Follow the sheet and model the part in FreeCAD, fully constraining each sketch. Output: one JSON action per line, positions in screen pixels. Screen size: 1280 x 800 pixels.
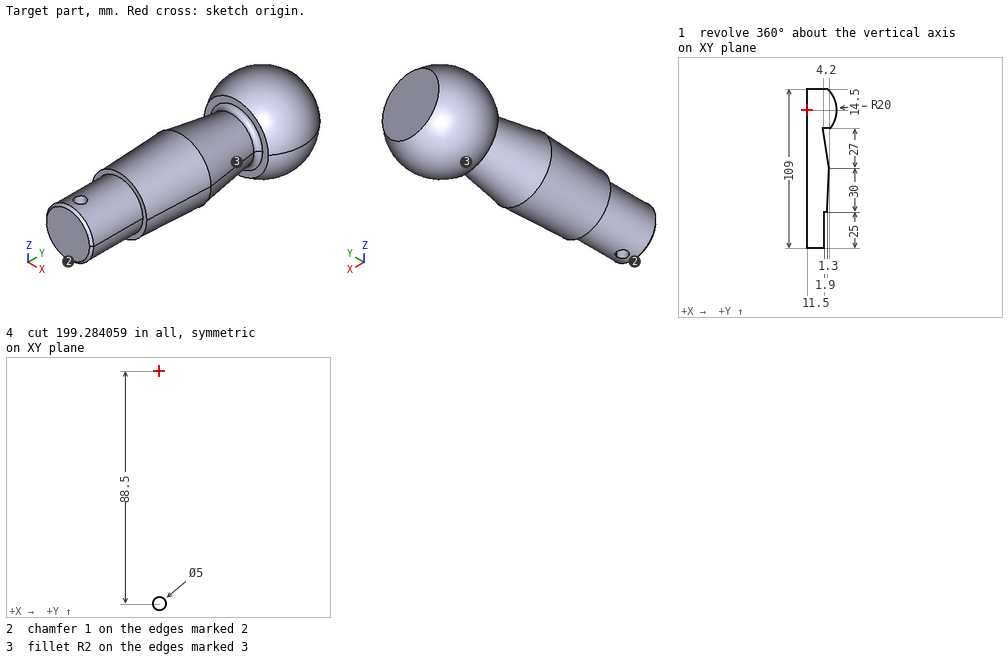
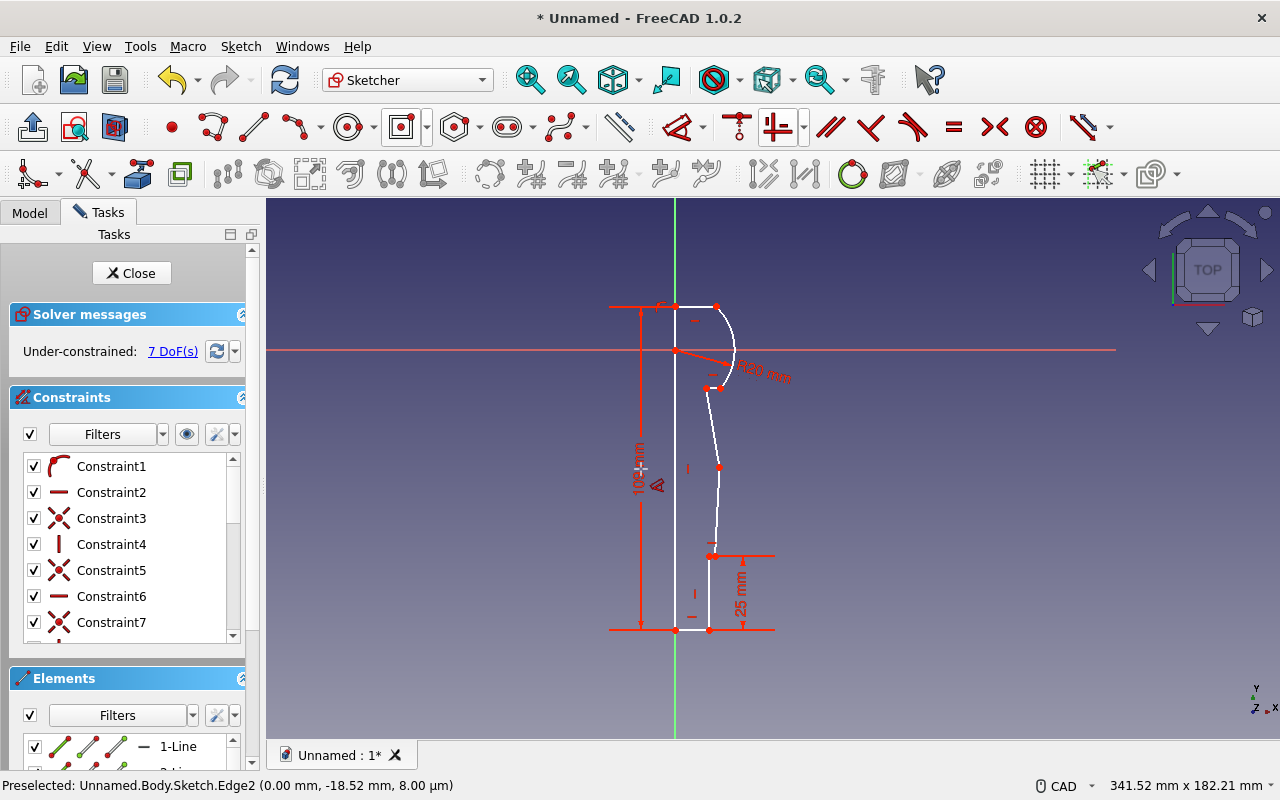
{"action": "scroll", "coordinate": [712, 556], "scroll_direction": "up", "scroll_amount": 10}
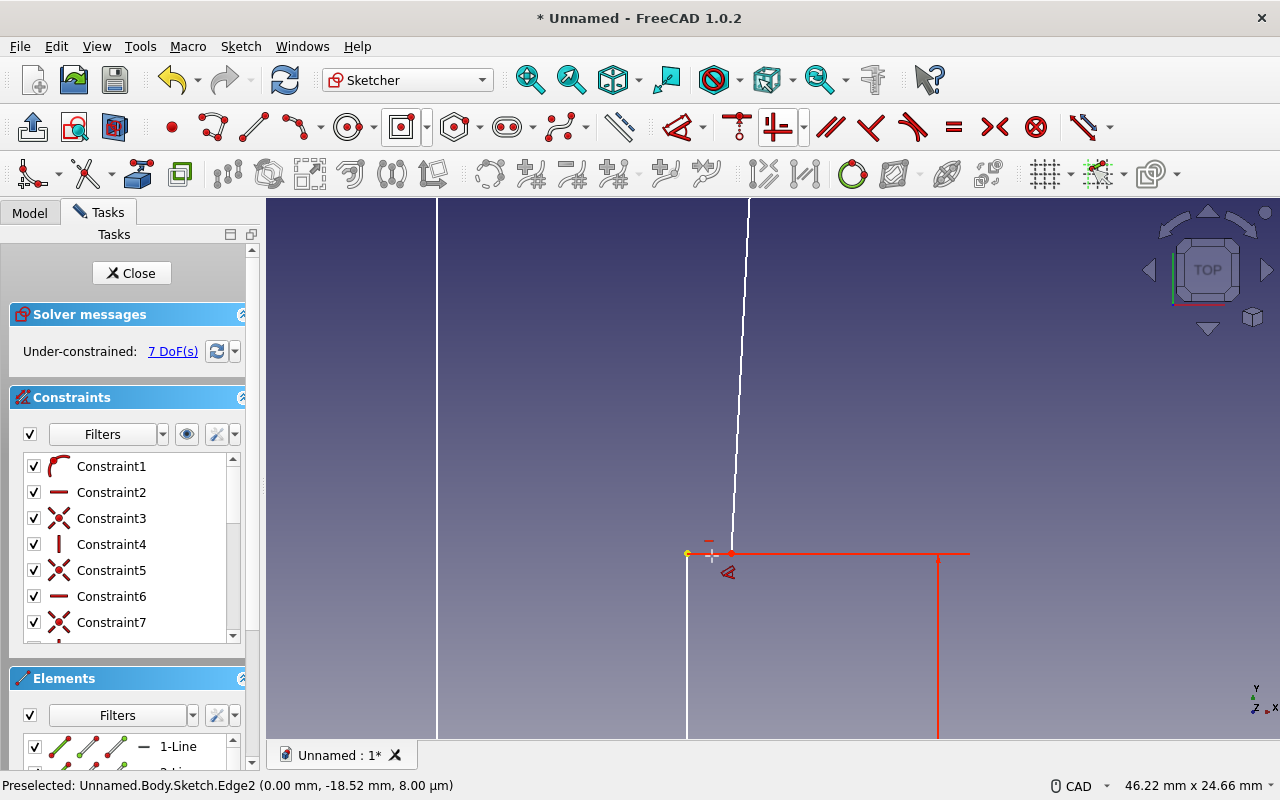
{"action": "left_click", "coordinate": [709, 554]}
{"action": "left_click", "coordinate": [709, 588]}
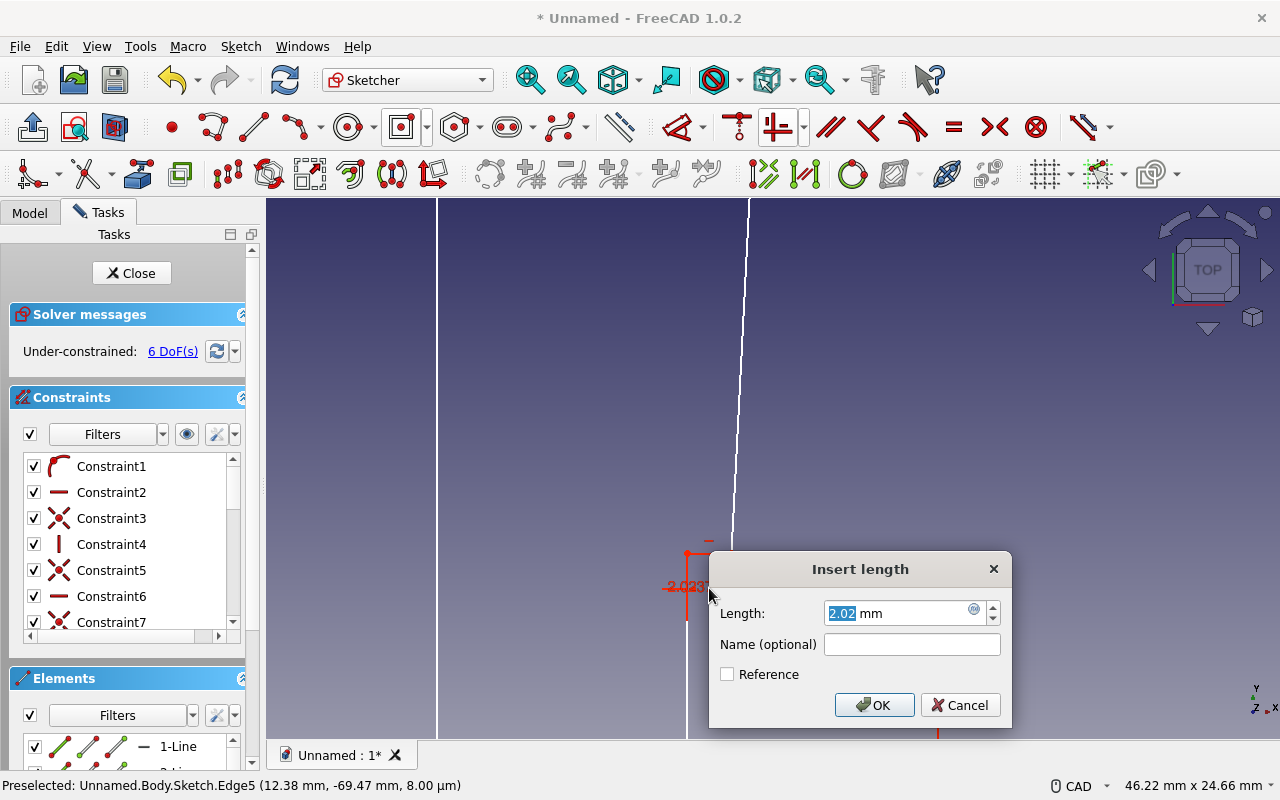
{"action": "type", "text": "1.9"}
{"action": "key", "text": "Return"}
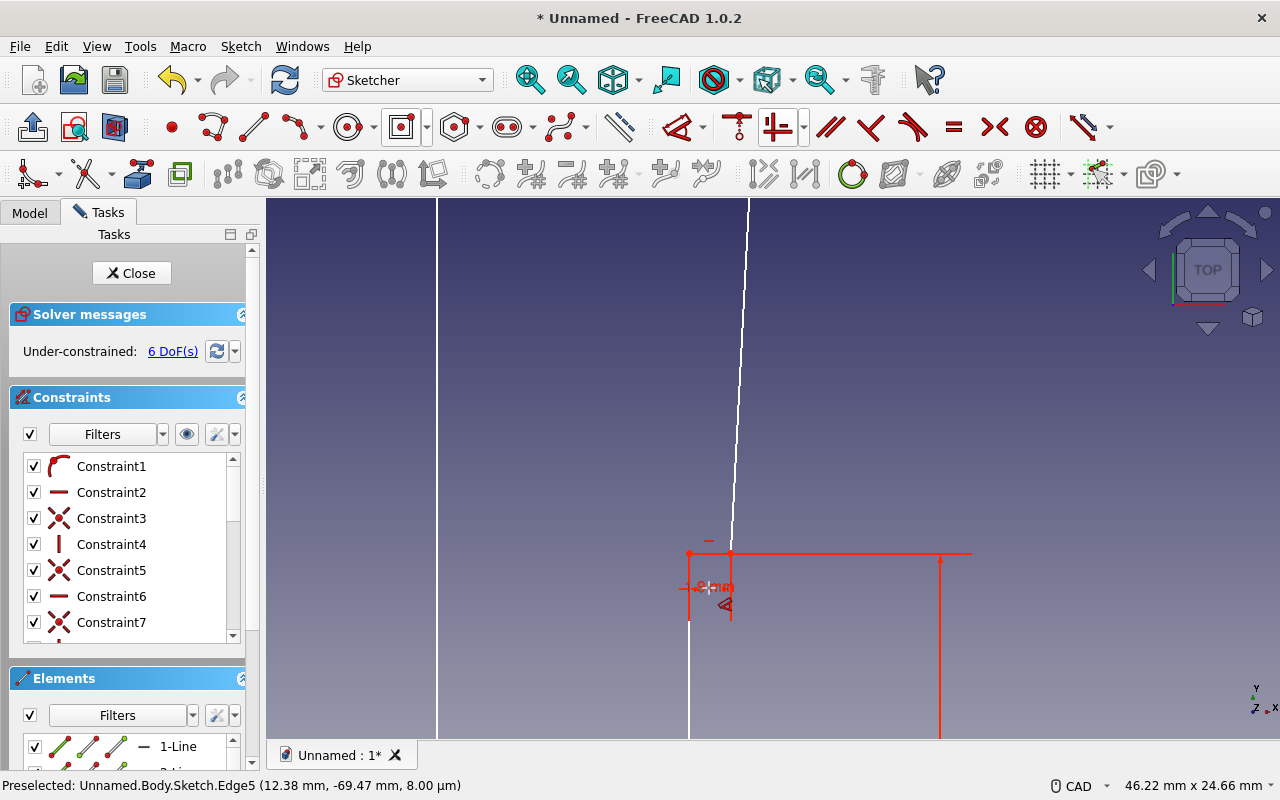
{"action": "scroll", "coordinate": [712, 556], "scroll_direction": "down", "scroll_amount": 10}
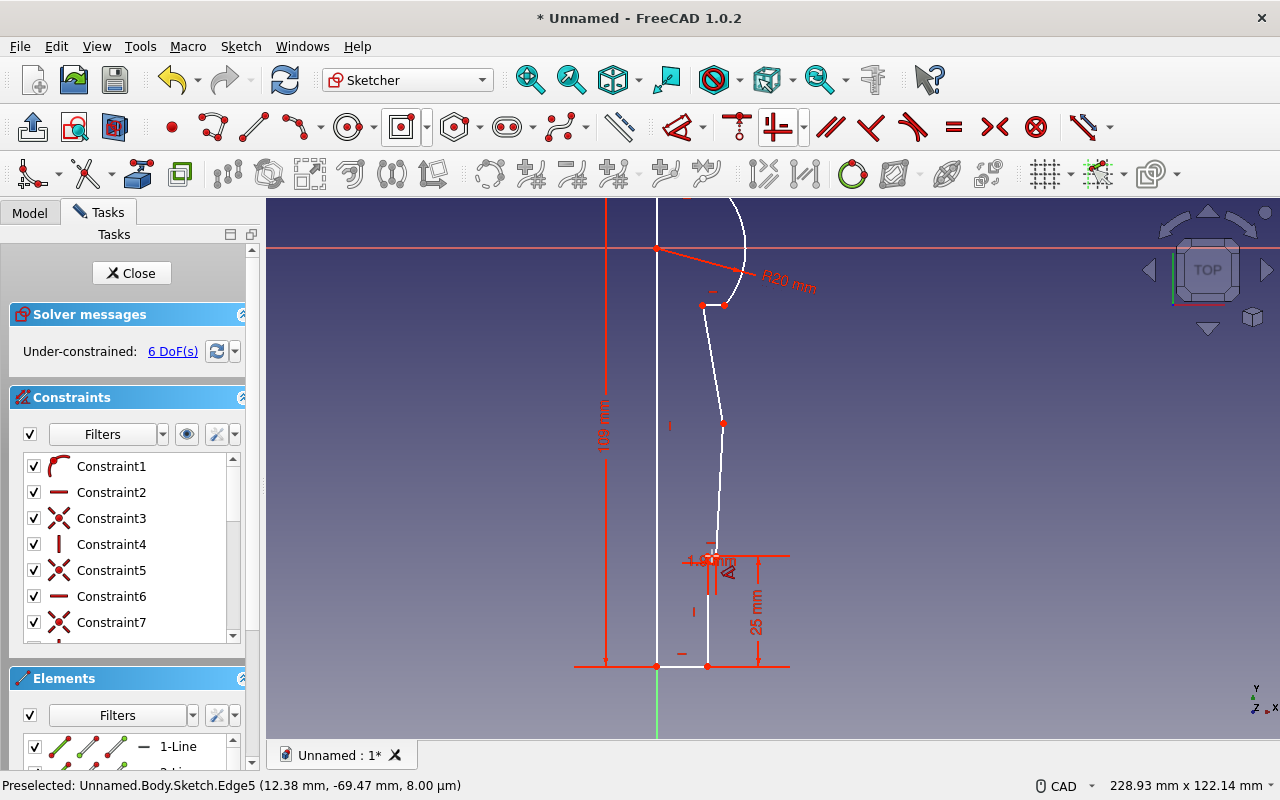
{"action": "left_click", "coordinate": [716, 530]}
{"action": "left_click", "coordinate": [754, 512]}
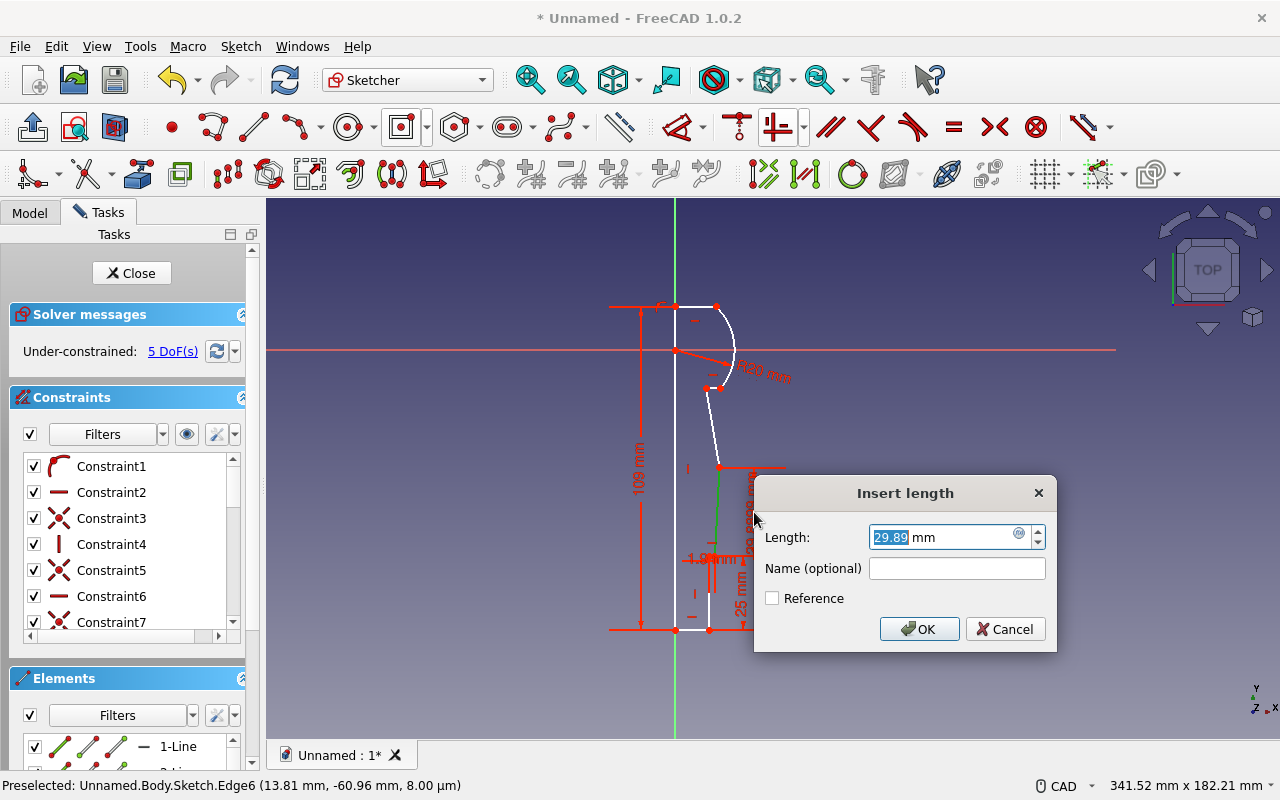
{"action": "type", "text": "30"}
{"action": "key", "text": "Return"}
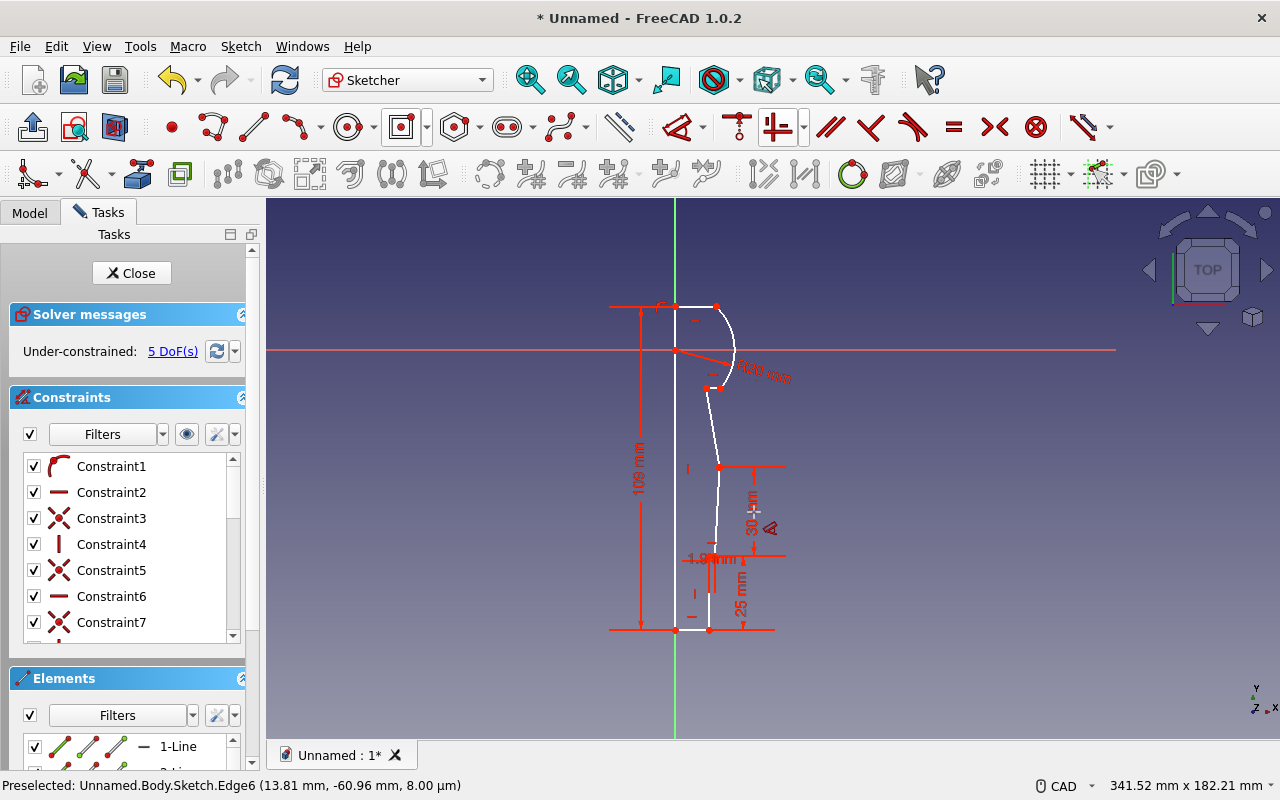
{"action": "left_click", "coordinate": [715, 443]}
{"action": "left_click", "coordinate": [754, 428]}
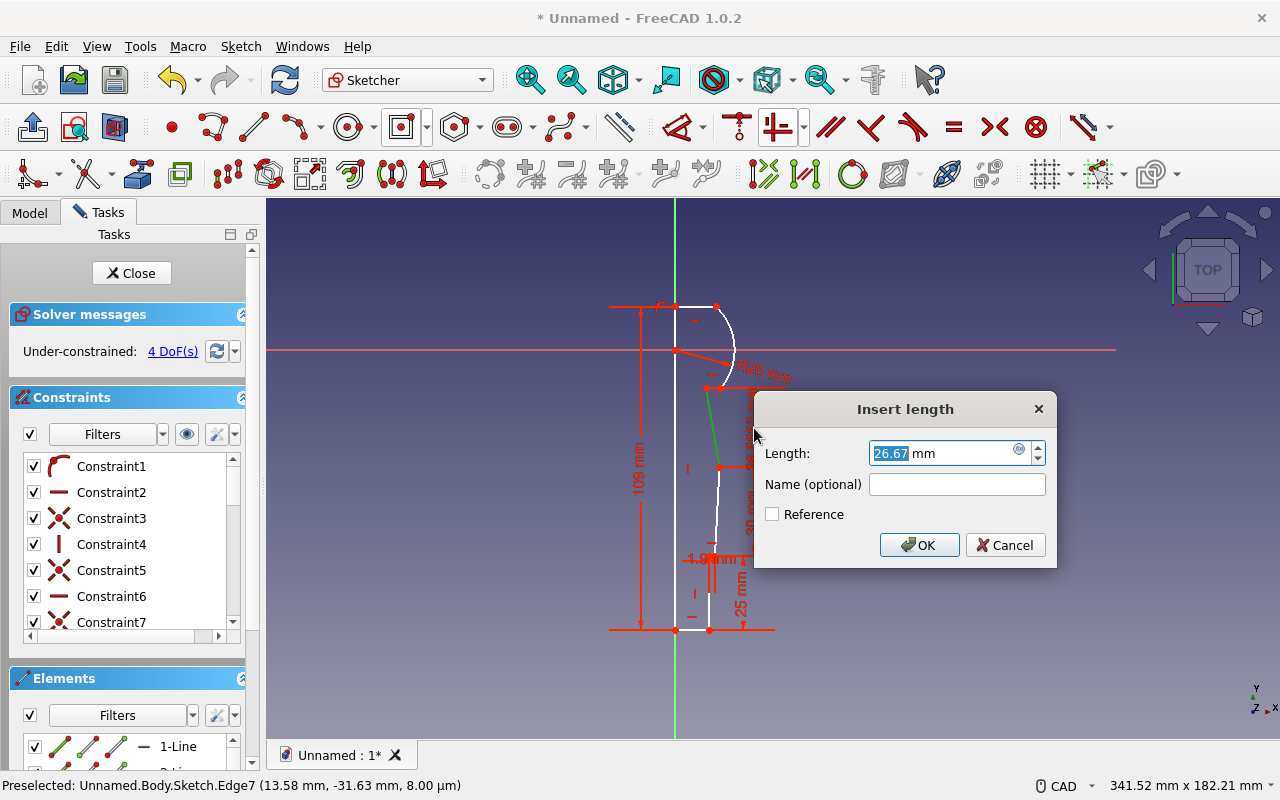
{"action": "type", "text": "27"}
{"action": "key", "text": "Return"}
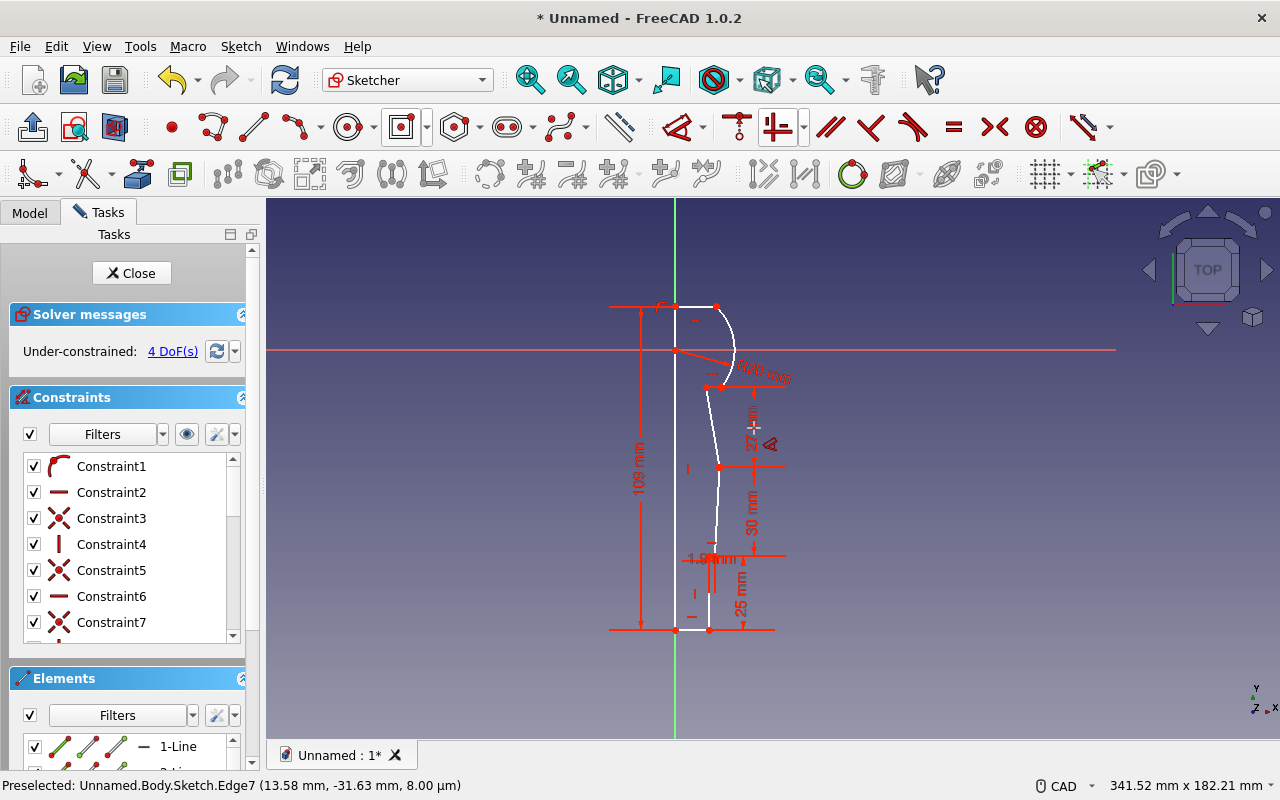
{"action": "scroll", "coordinate": [685, 630], "scroll_direction": "up", "scroll_amount": 2}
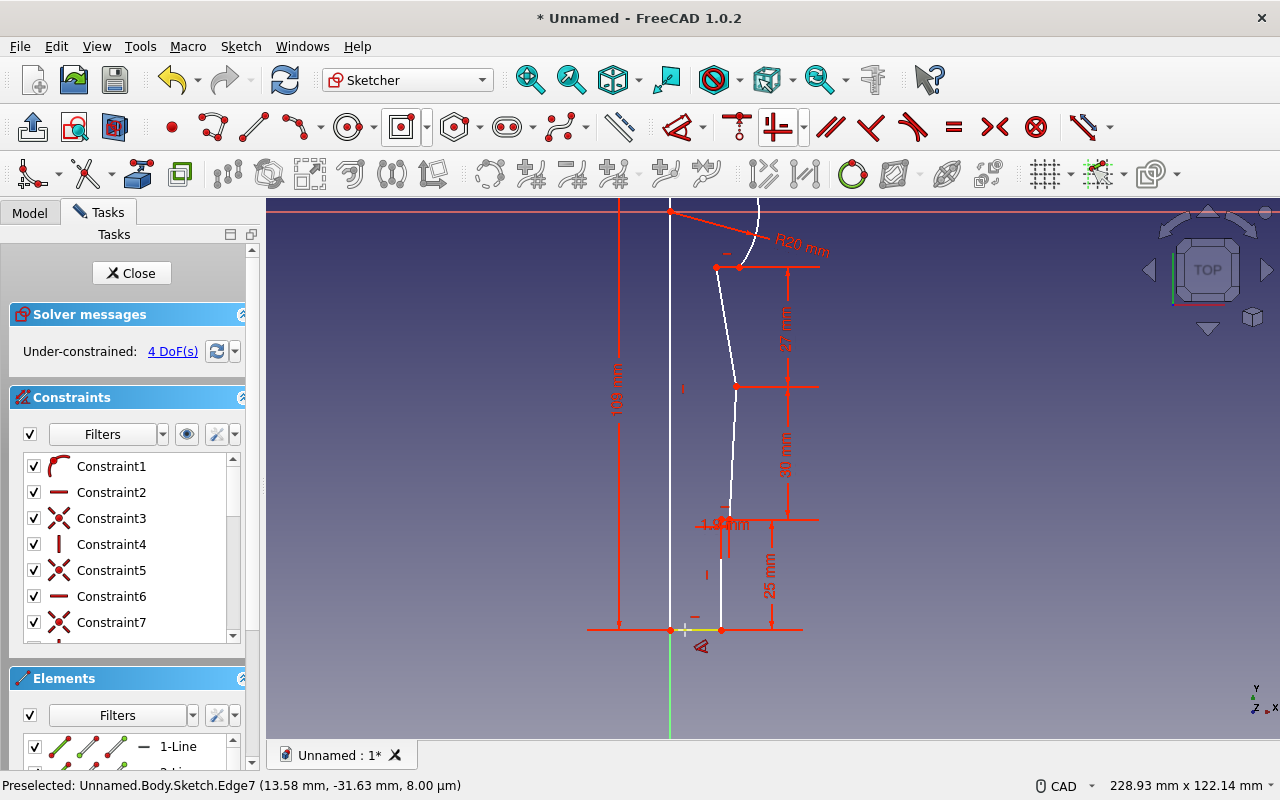
{"action": "left_click", "coordinate": [685, 630]}
{"action": "left_click", "coordinate": [696, 664]}